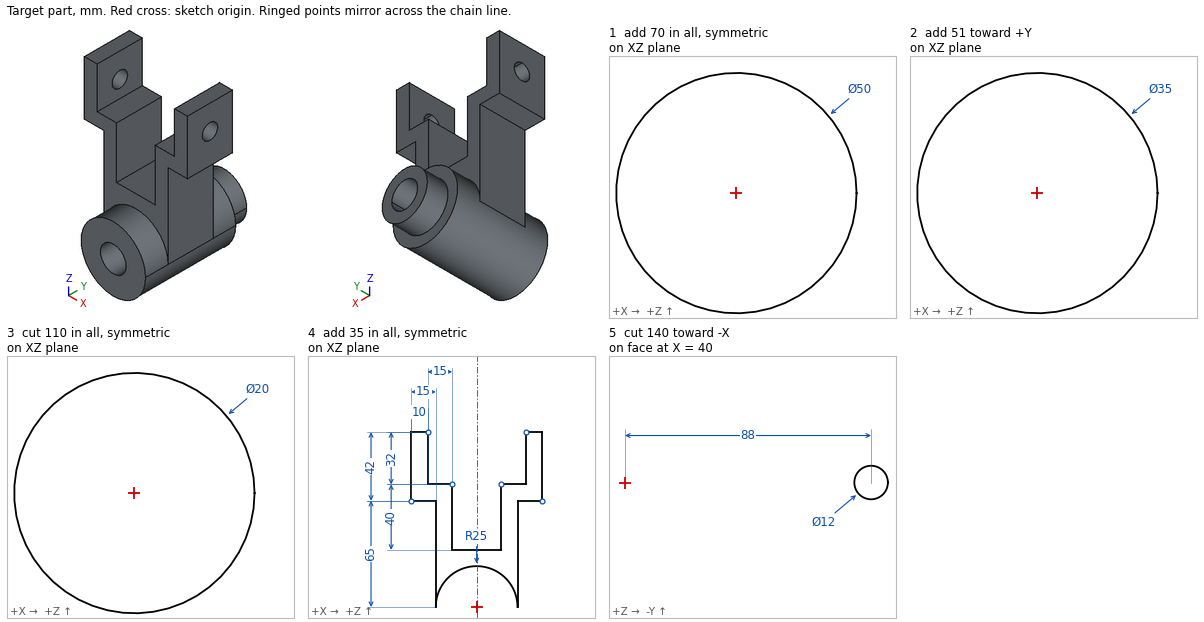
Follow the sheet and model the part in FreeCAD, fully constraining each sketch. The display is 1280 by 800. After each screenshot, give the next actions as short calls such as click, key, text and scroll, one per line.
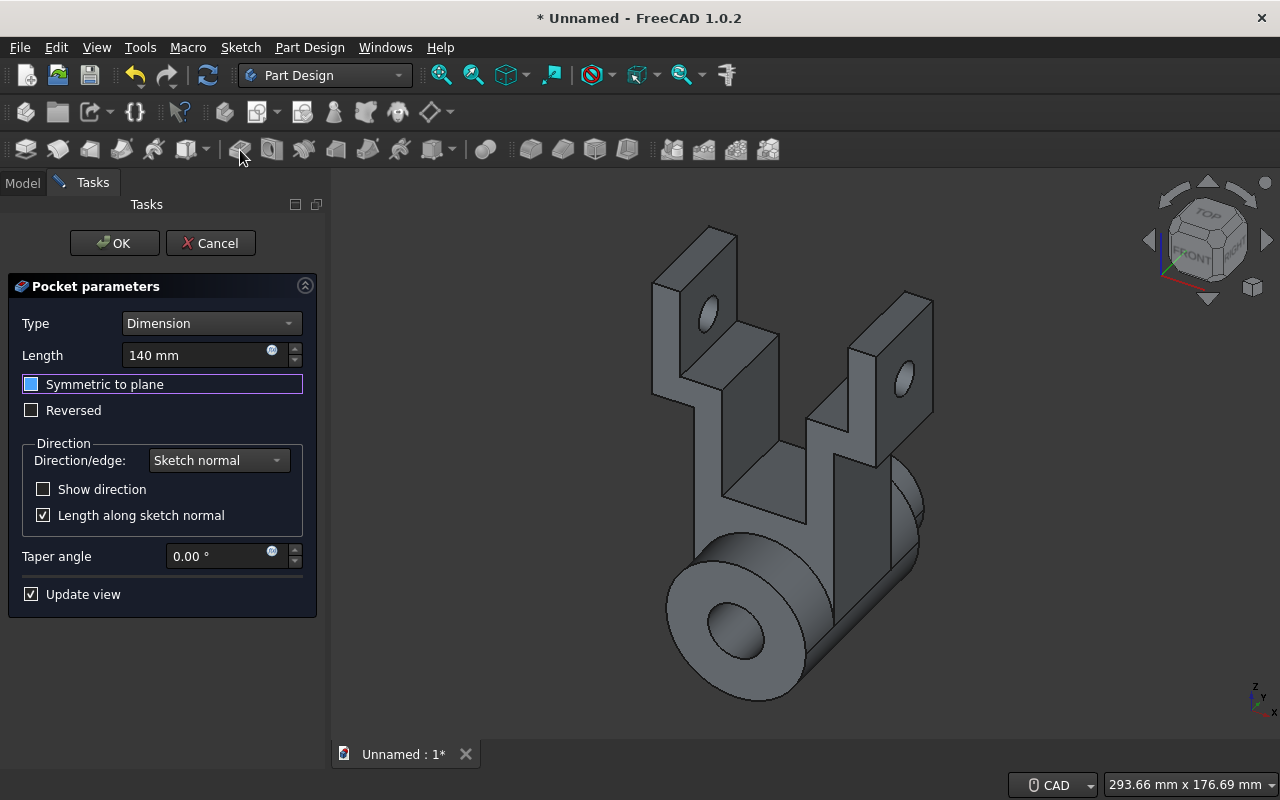
click(115, 243)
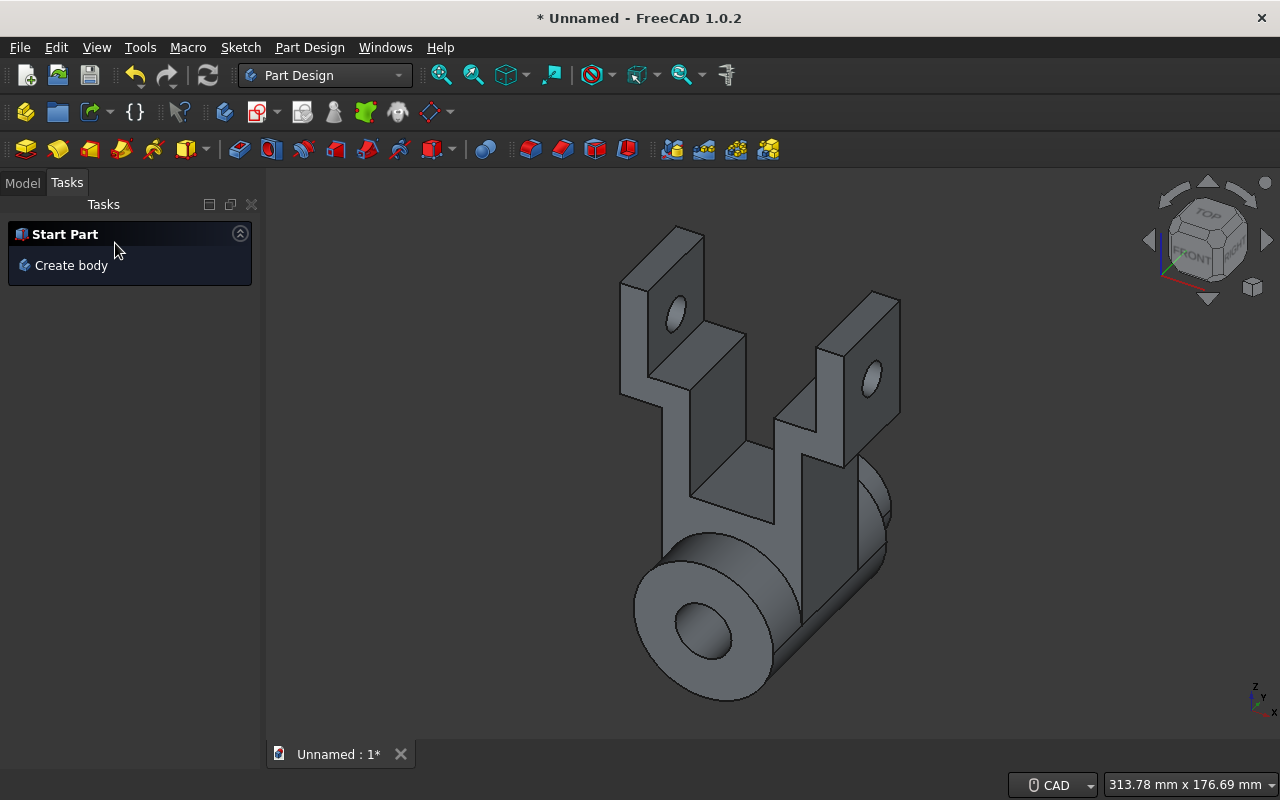
key(0)